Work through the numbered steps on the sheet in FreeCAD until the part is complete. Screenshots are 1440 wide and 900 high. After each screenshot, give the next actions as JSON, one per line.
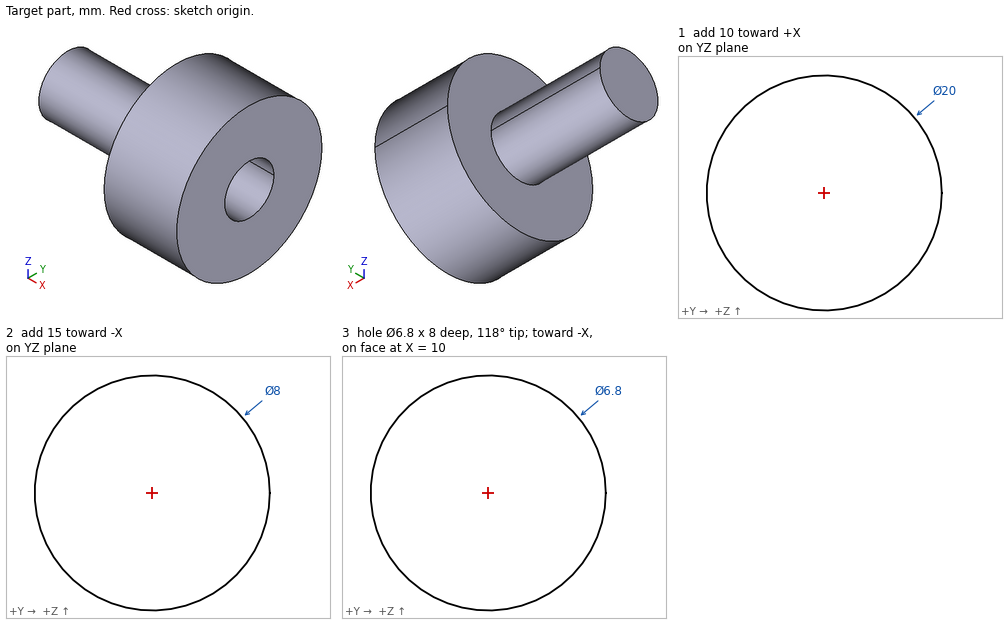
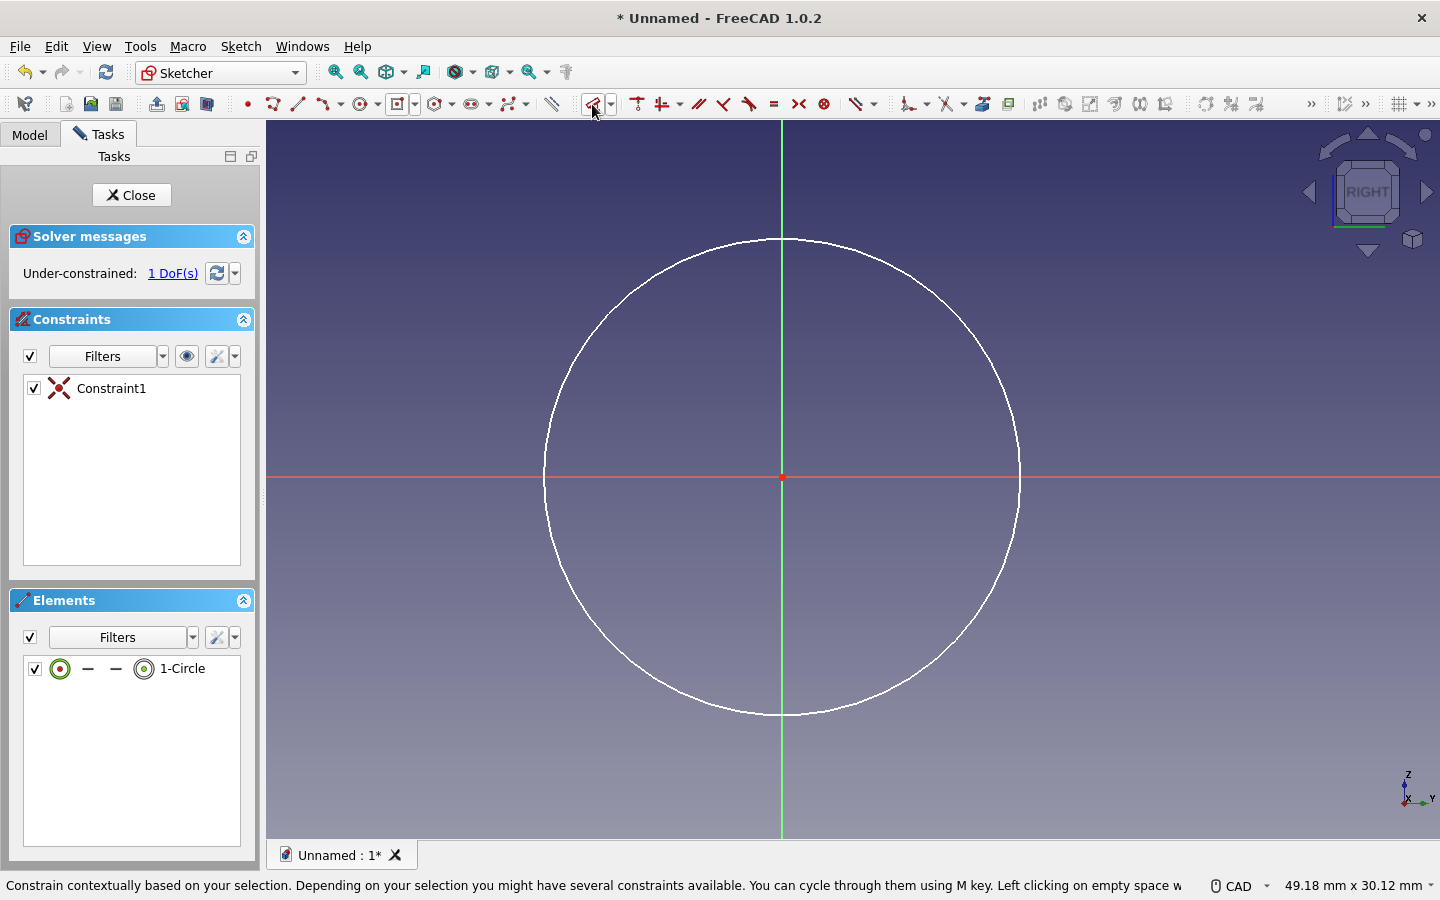
{"action": "left_click", "coordinate": [950, 308]}
{"action": "left_click", "coordinate": [973, 285]}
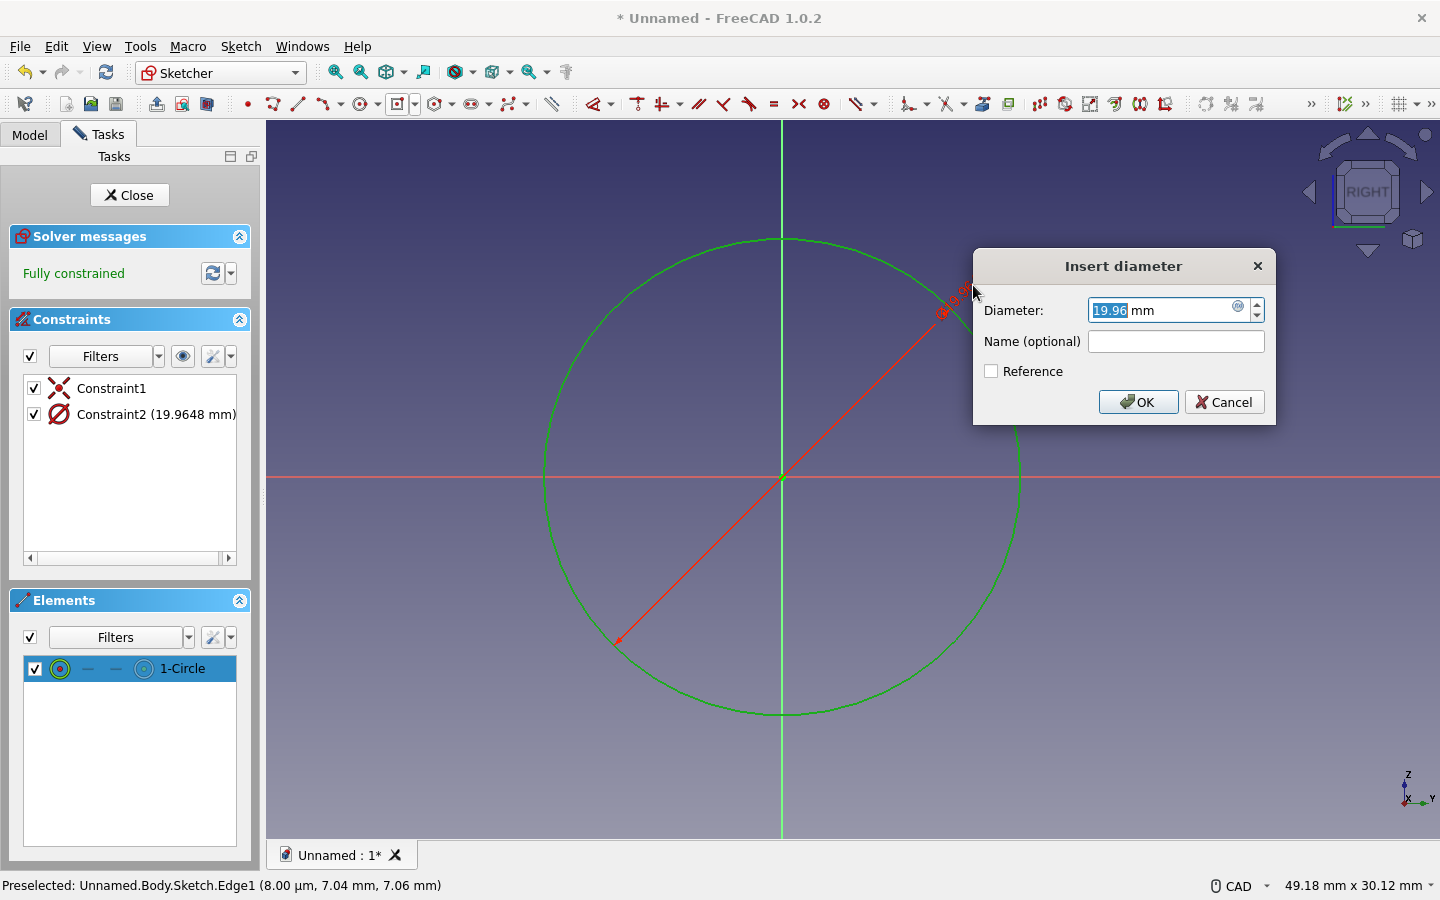
{"action": "type", "text": "20"}
{"action": "key", "text": "Return"}
{"action": "key", "text": "Escape"}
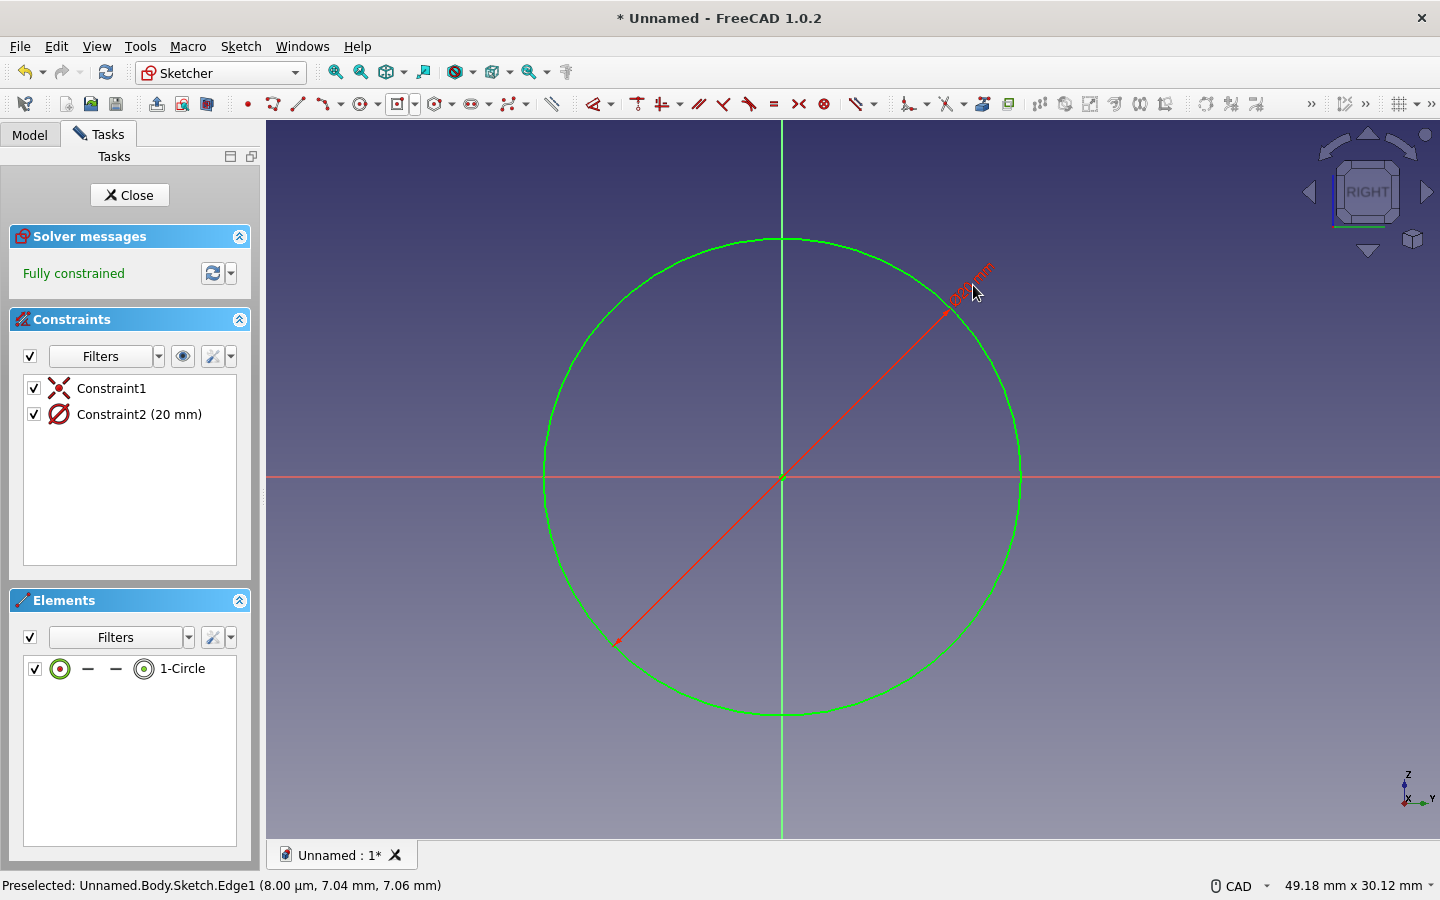
{"action": "left_click", "coordinate": [130, 195]}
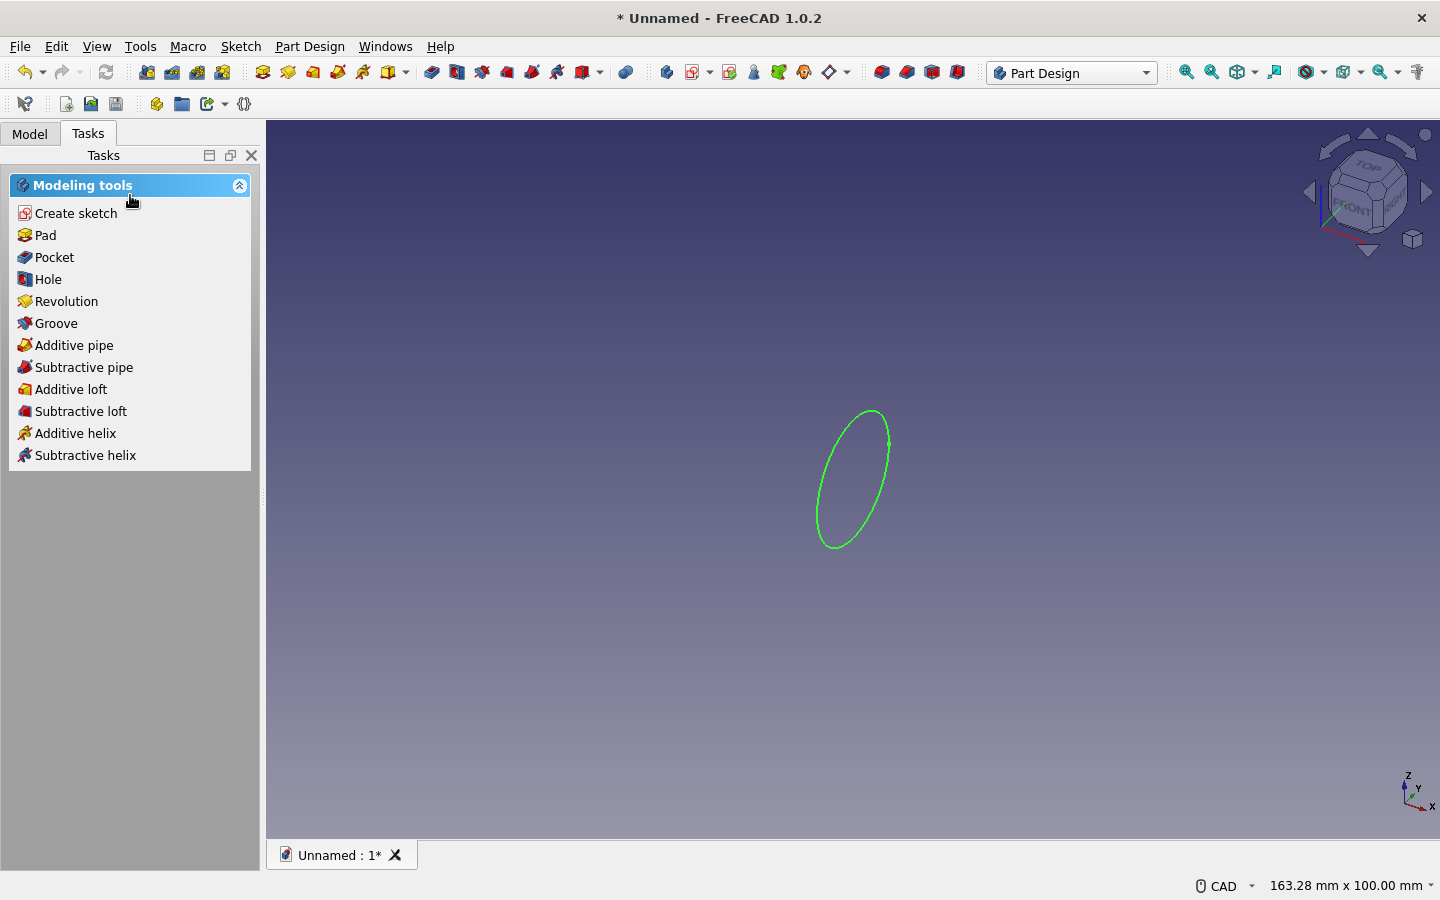
{"action": "left_click", "coordinate": [263, 72]}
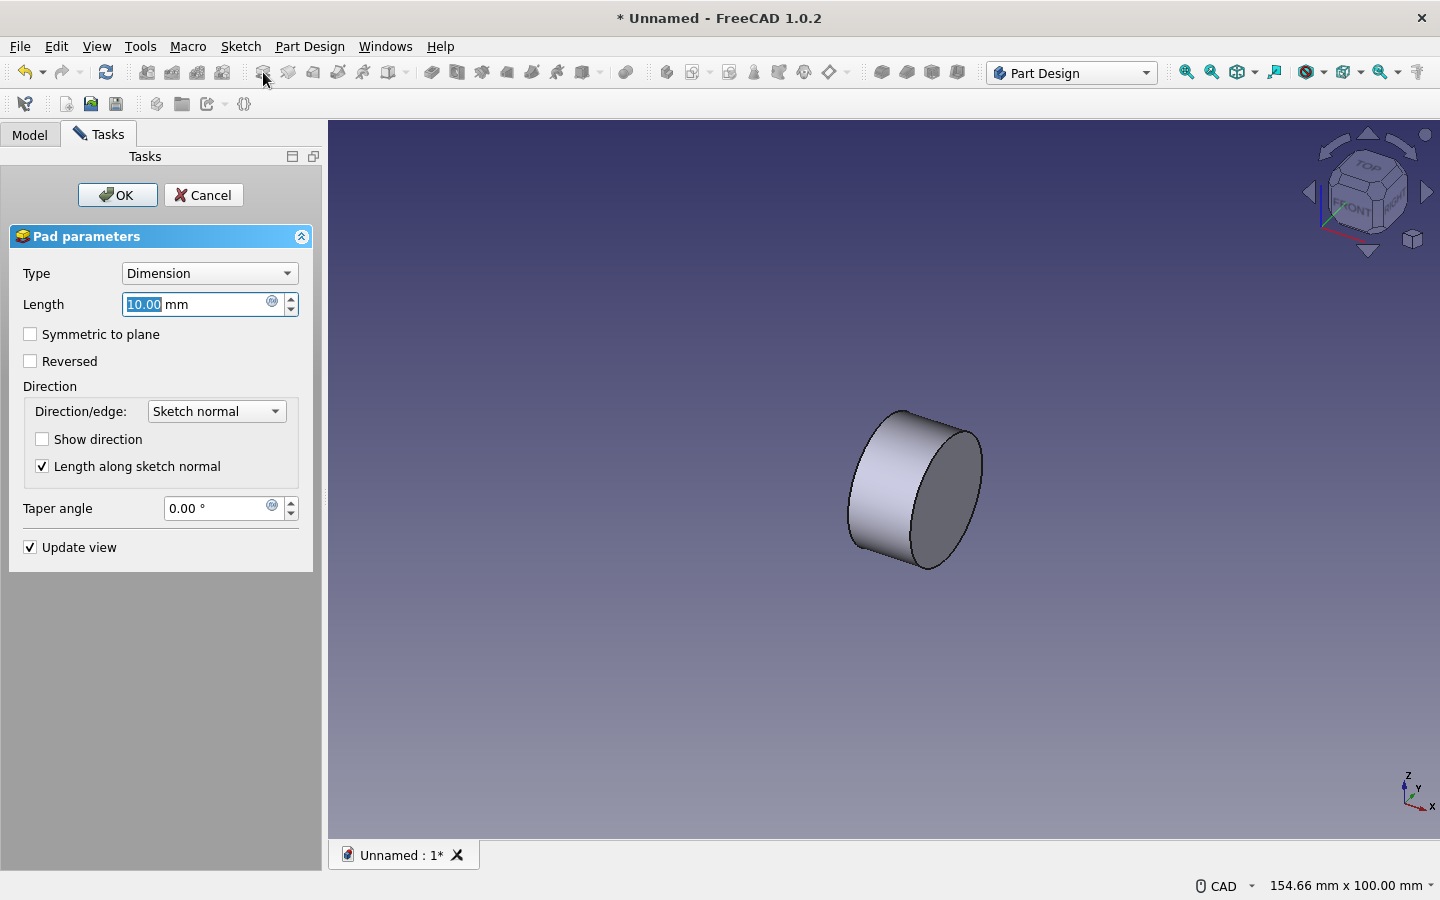
{"action": "type", "text": "10"}
{"action": "key", "text": "Tab"}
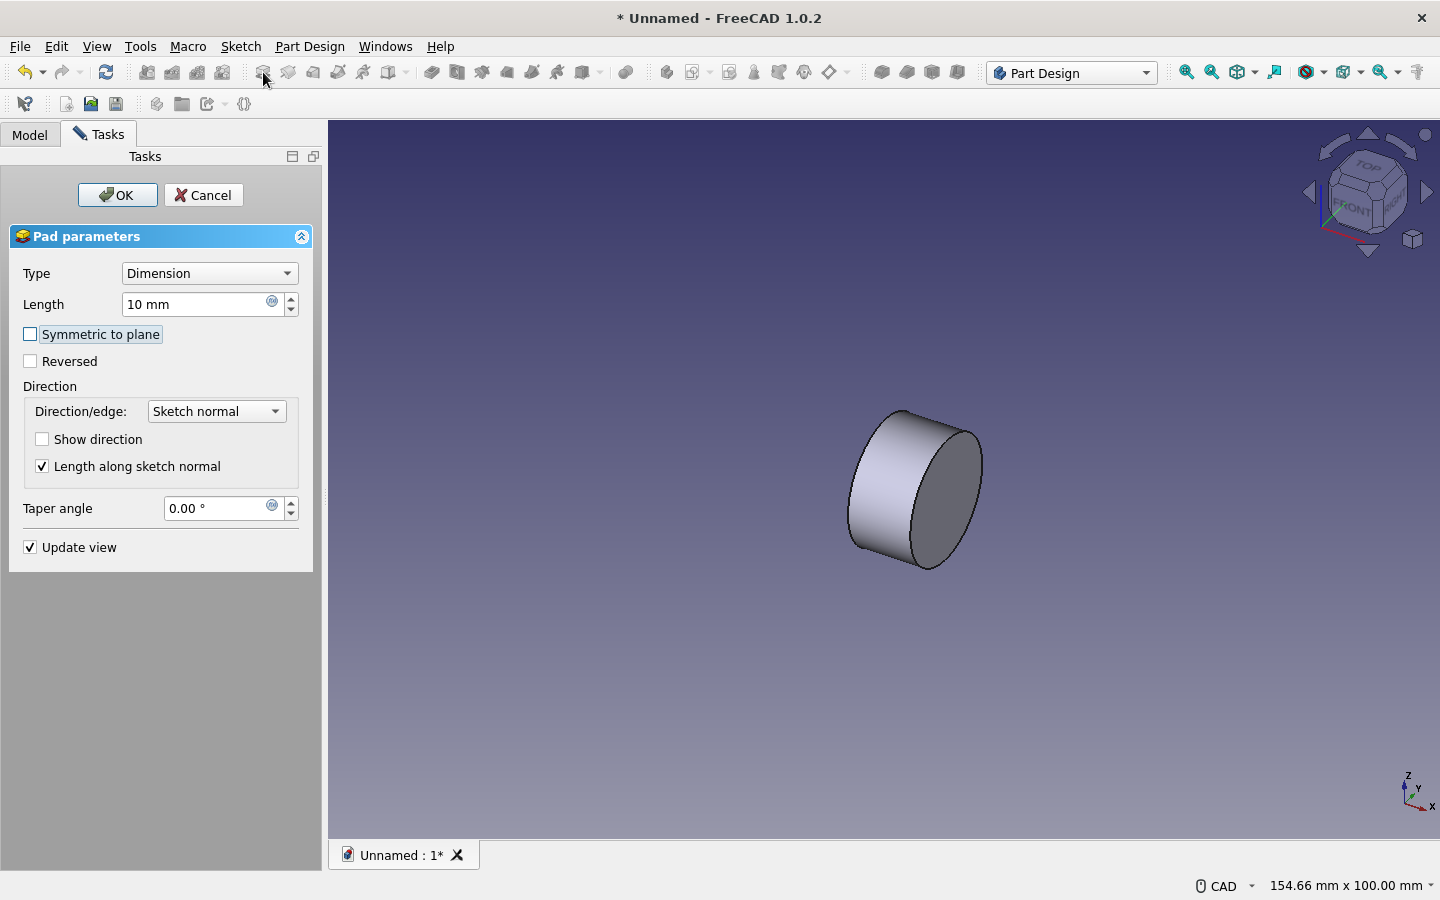
{"action": "left_click", "coordinate": [118, 195]}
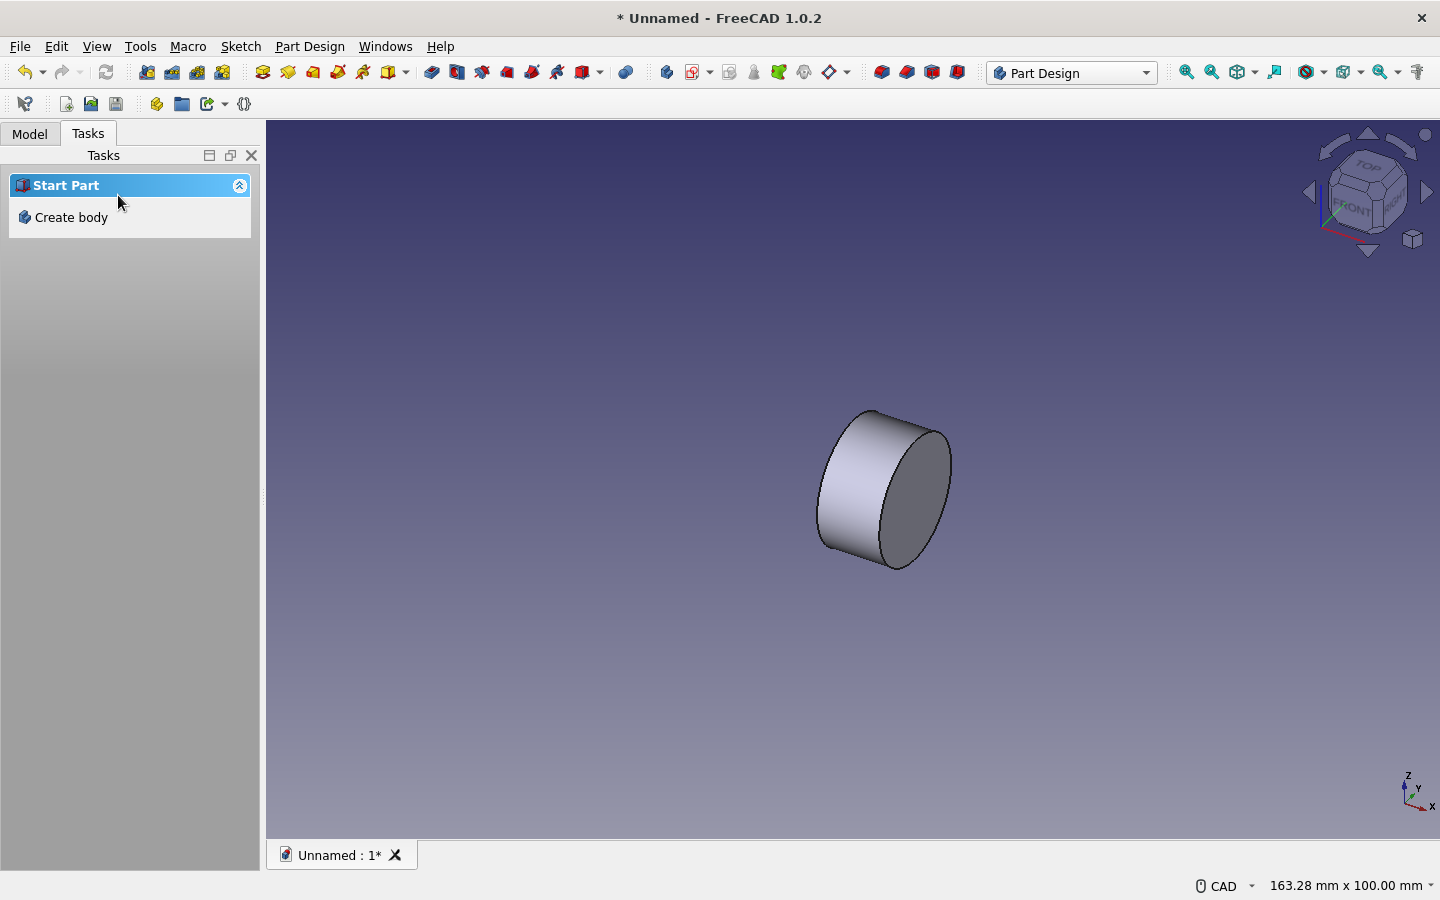
{"action": "left_click", "coordinate": [1187, 72]}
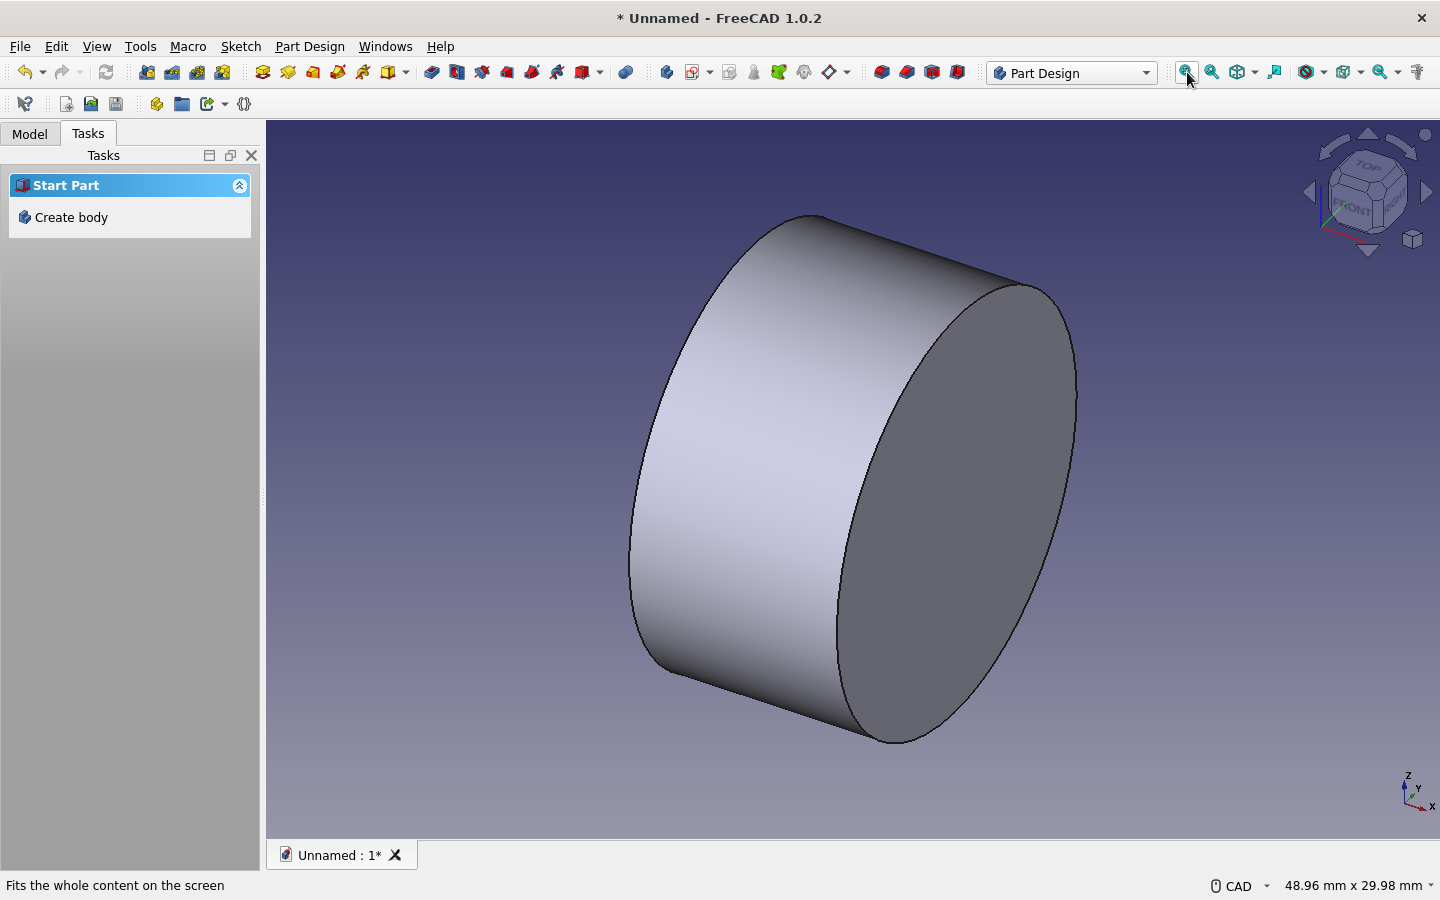
{"action": "left_click", "coordinate": [692, 72]}